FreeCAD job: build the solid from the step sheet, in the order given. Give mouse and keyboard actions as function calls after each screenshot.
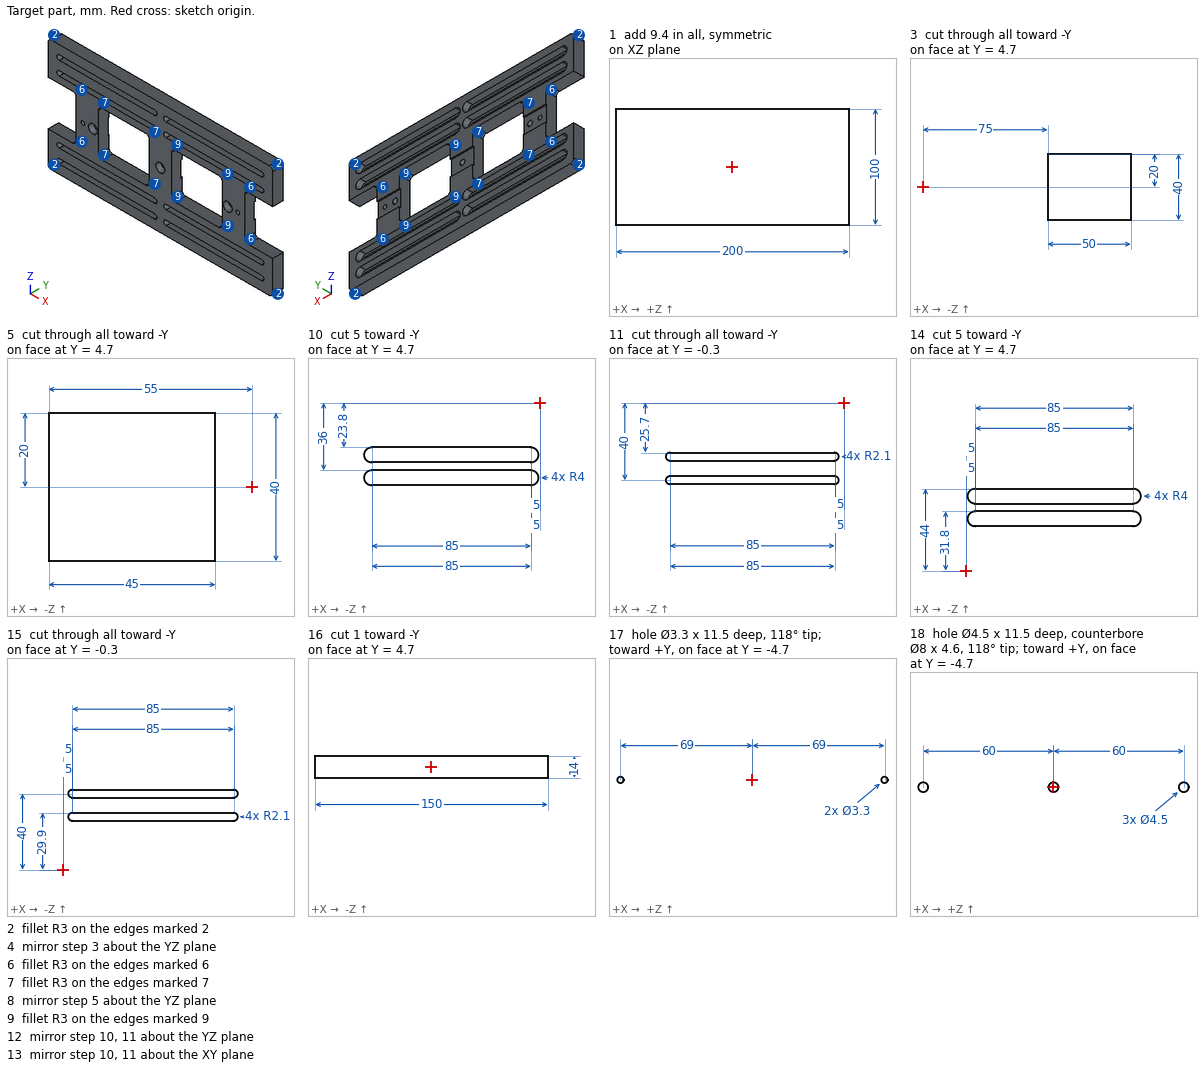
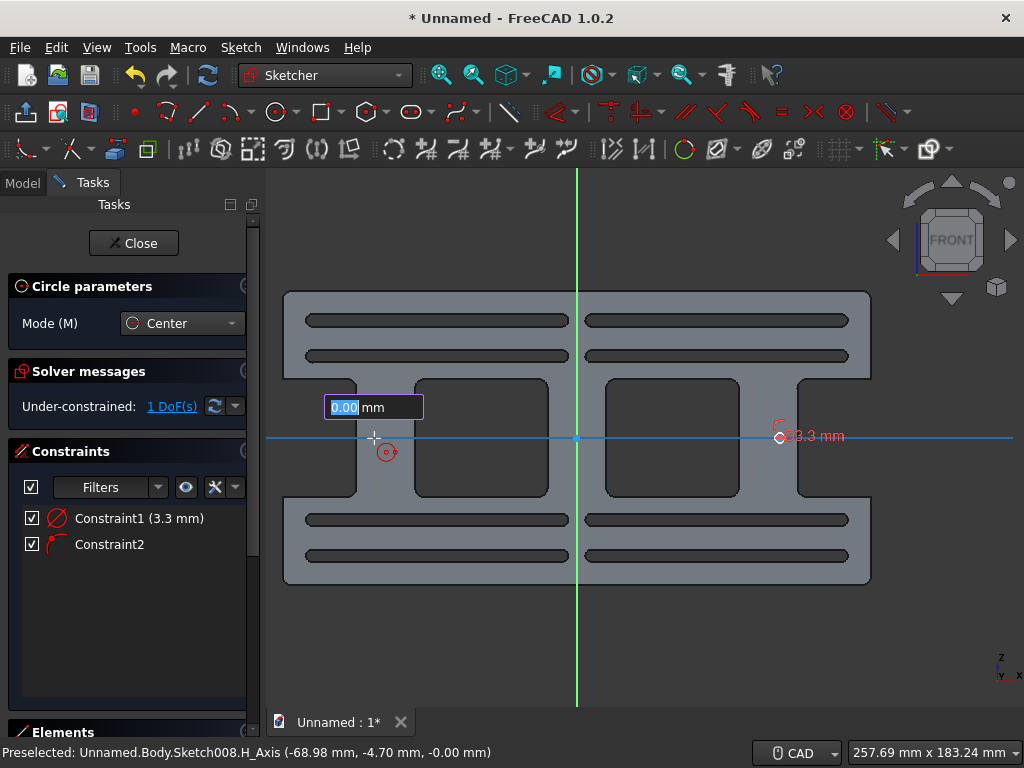
scroll(372, 443, up, 7)
move(373, 440)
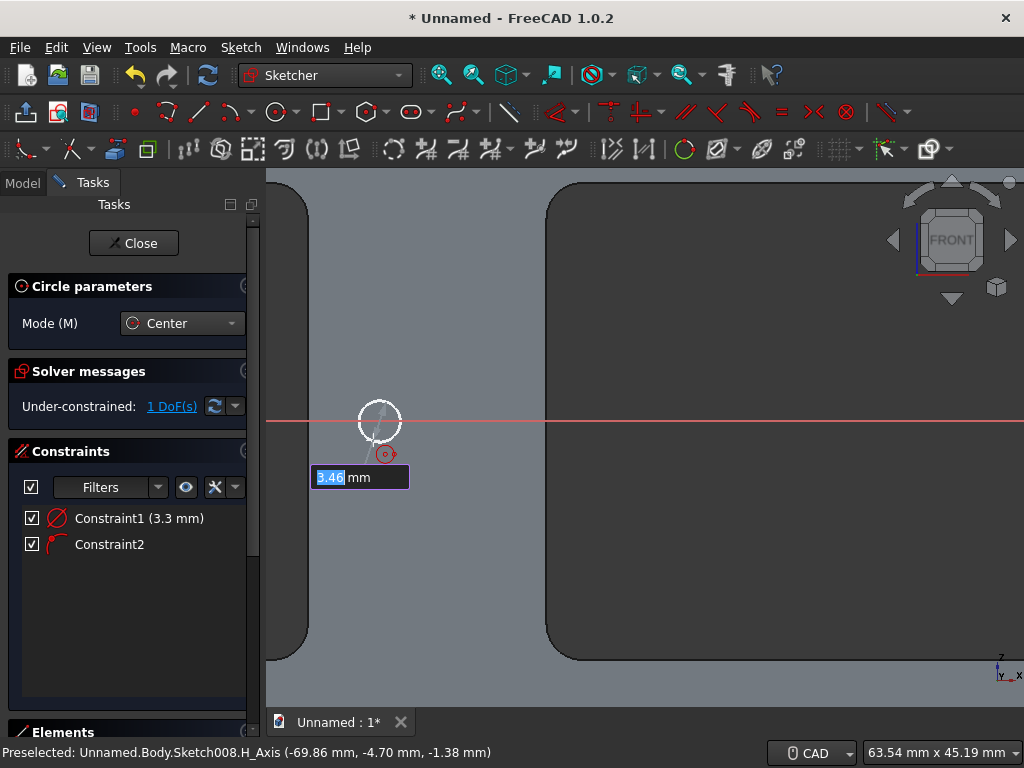
text(3.3)
key(Return)
key(Escape)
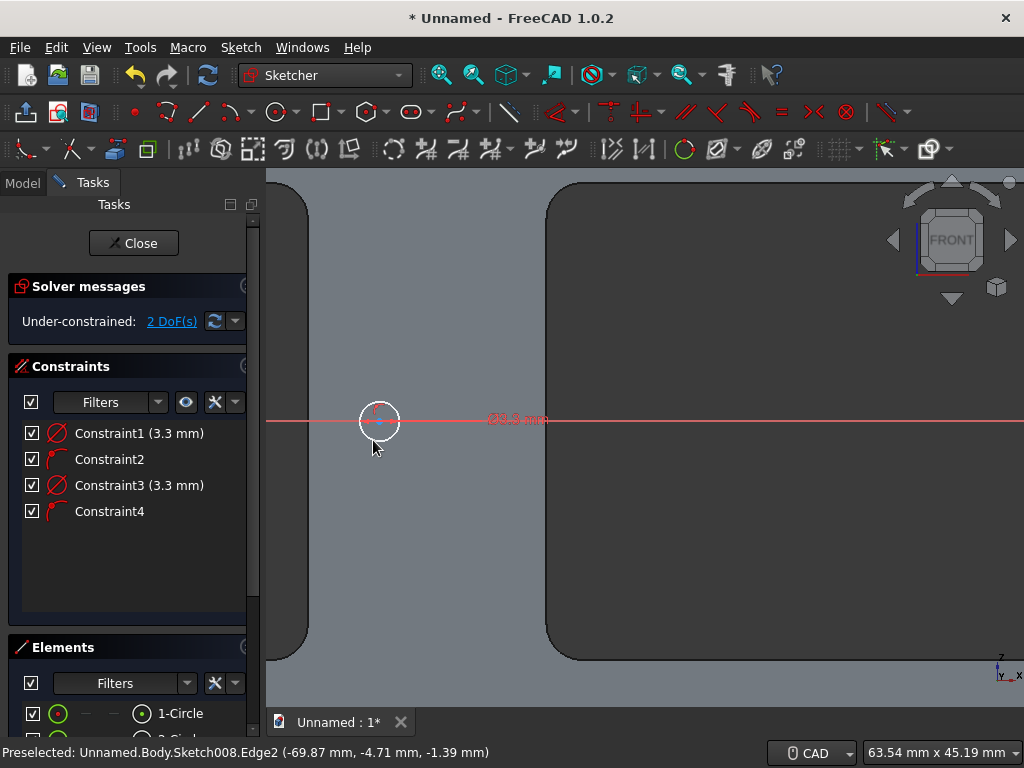
key(d)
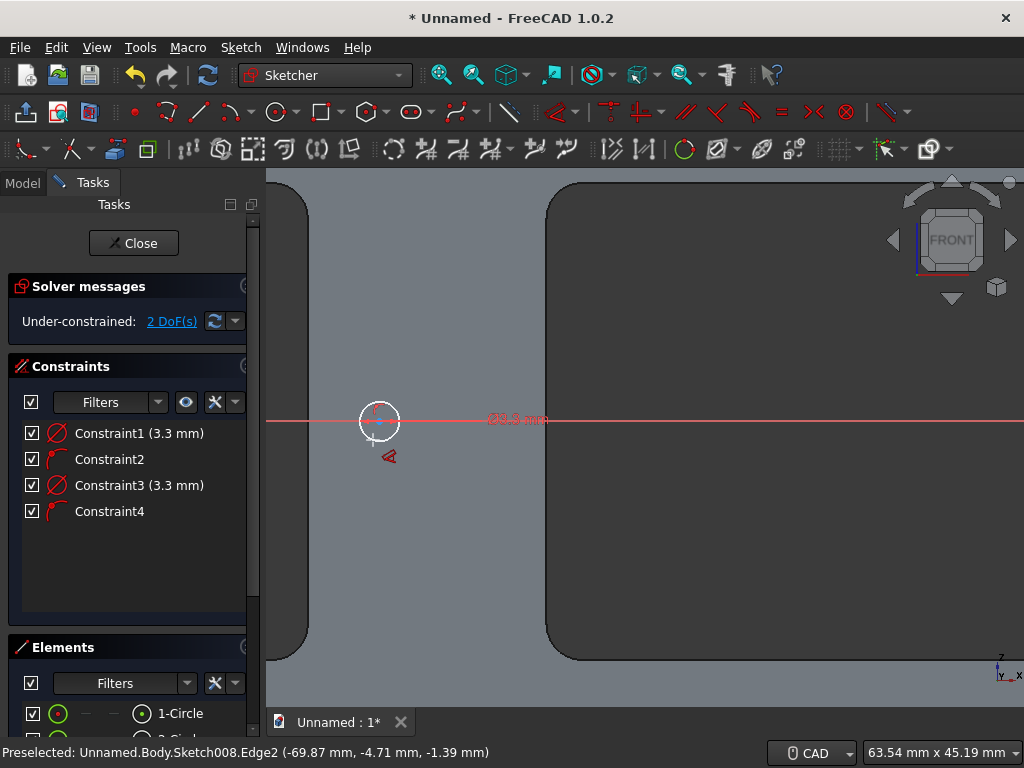
scroll(372, 443, down, 7)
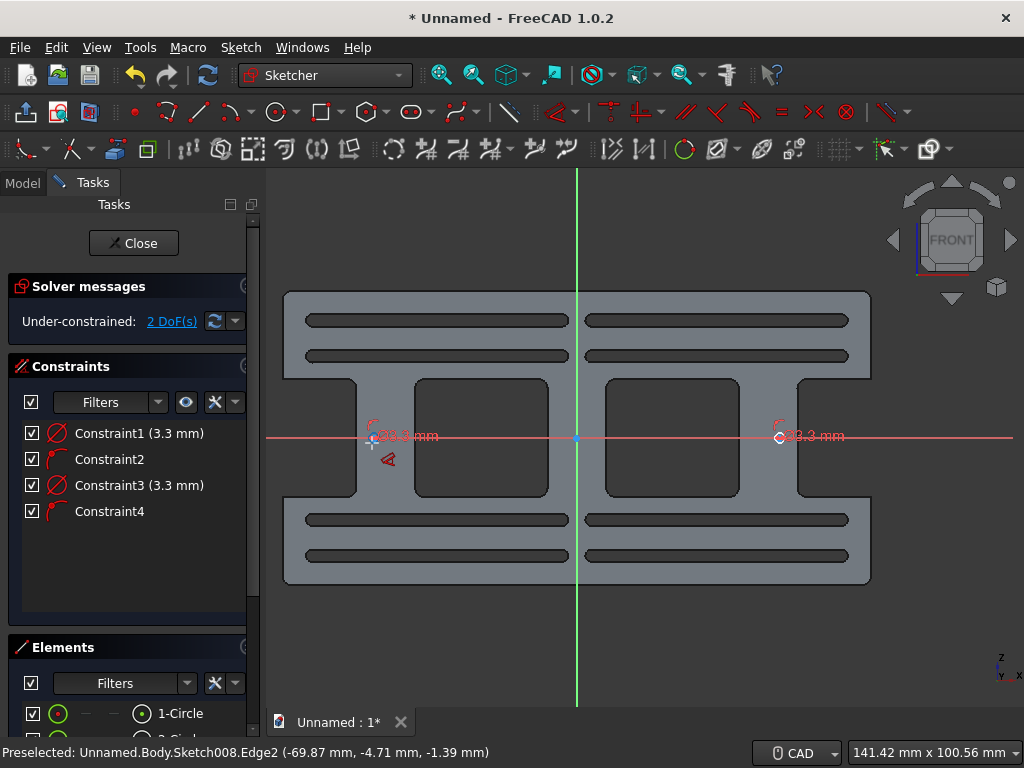
click(780, 438)
click(678, 472)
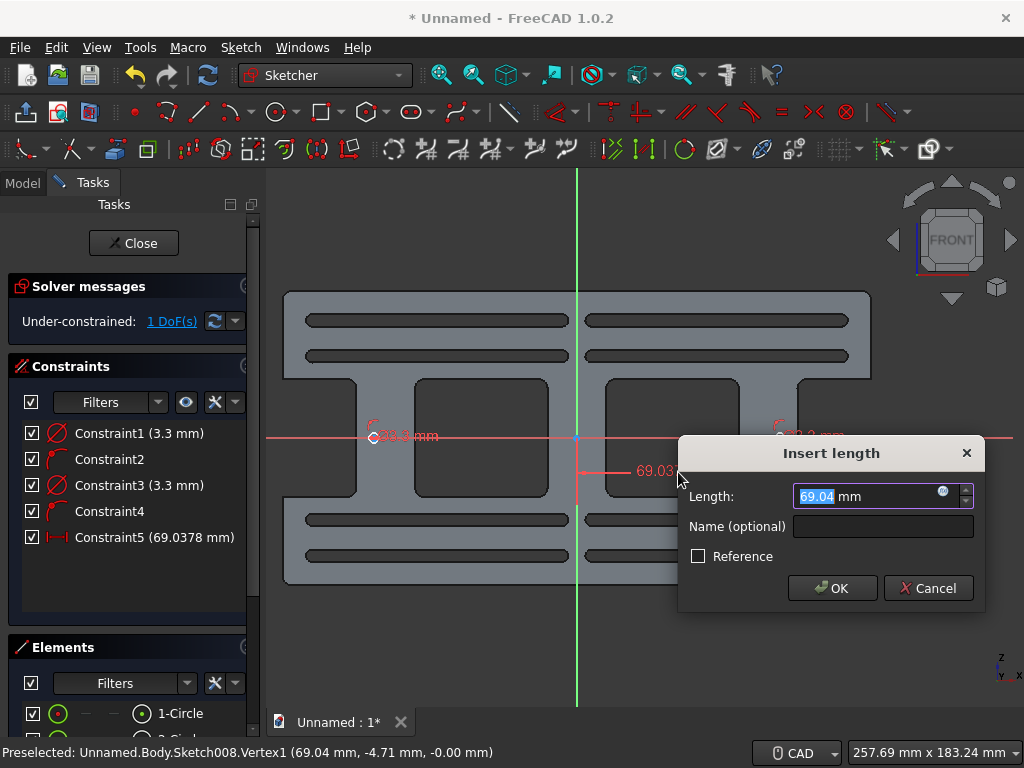
text(69)
key(Return)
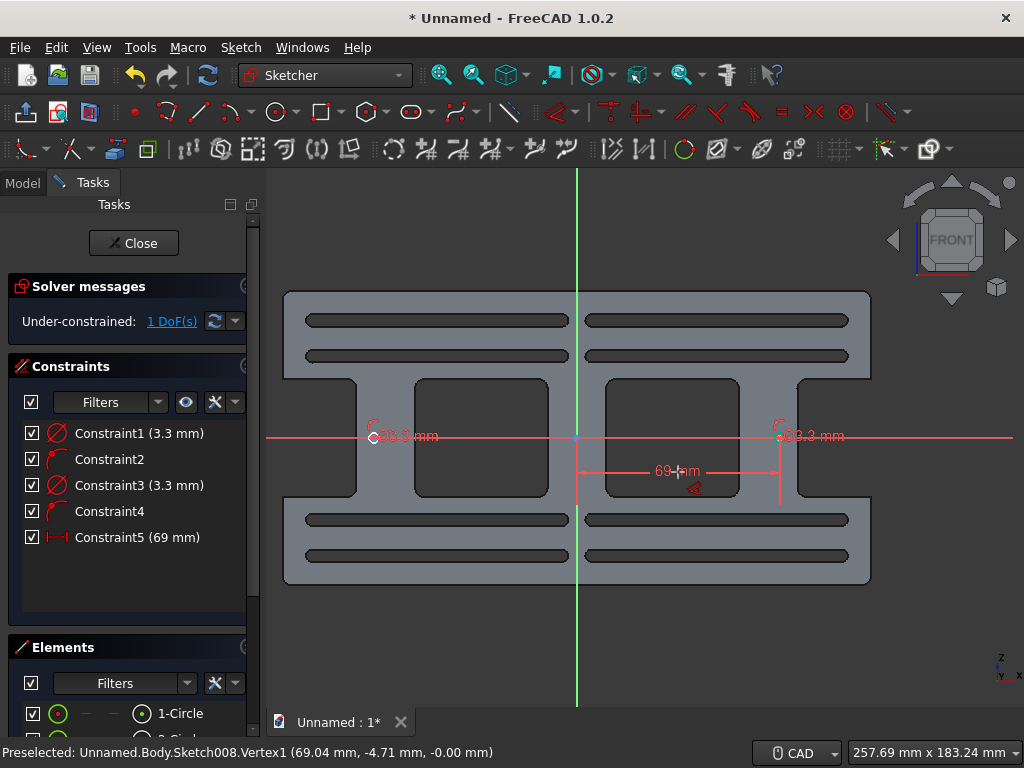
click(374, 438)
click(475, 472)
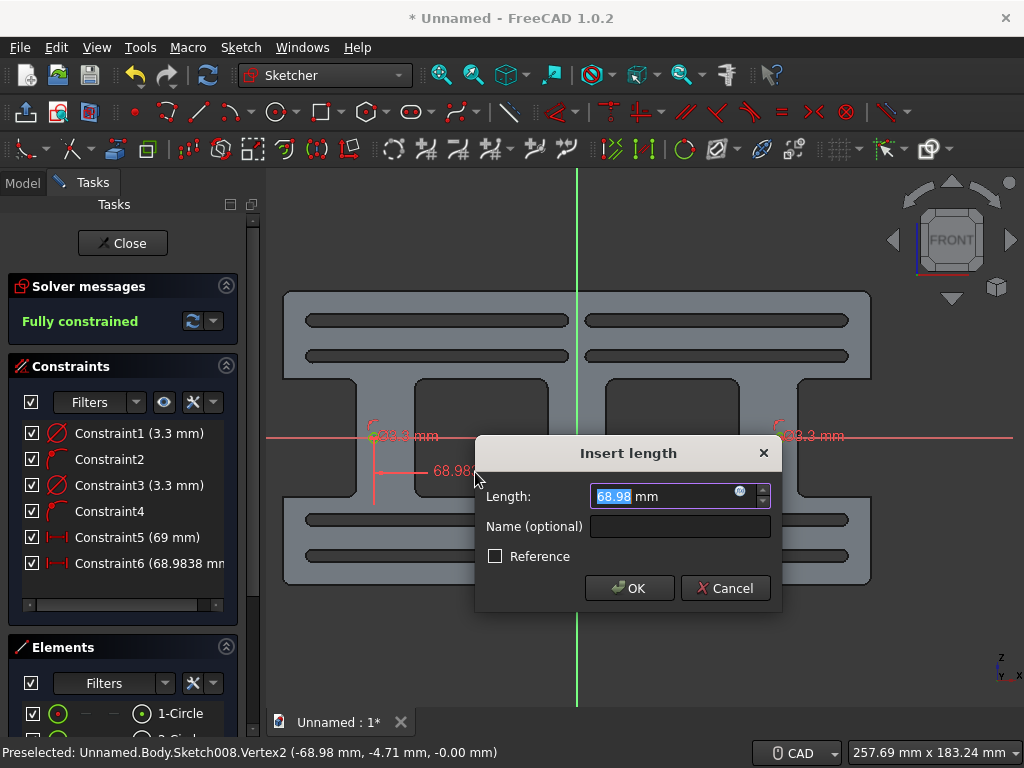
text(69)
key(Return)
key(Escape)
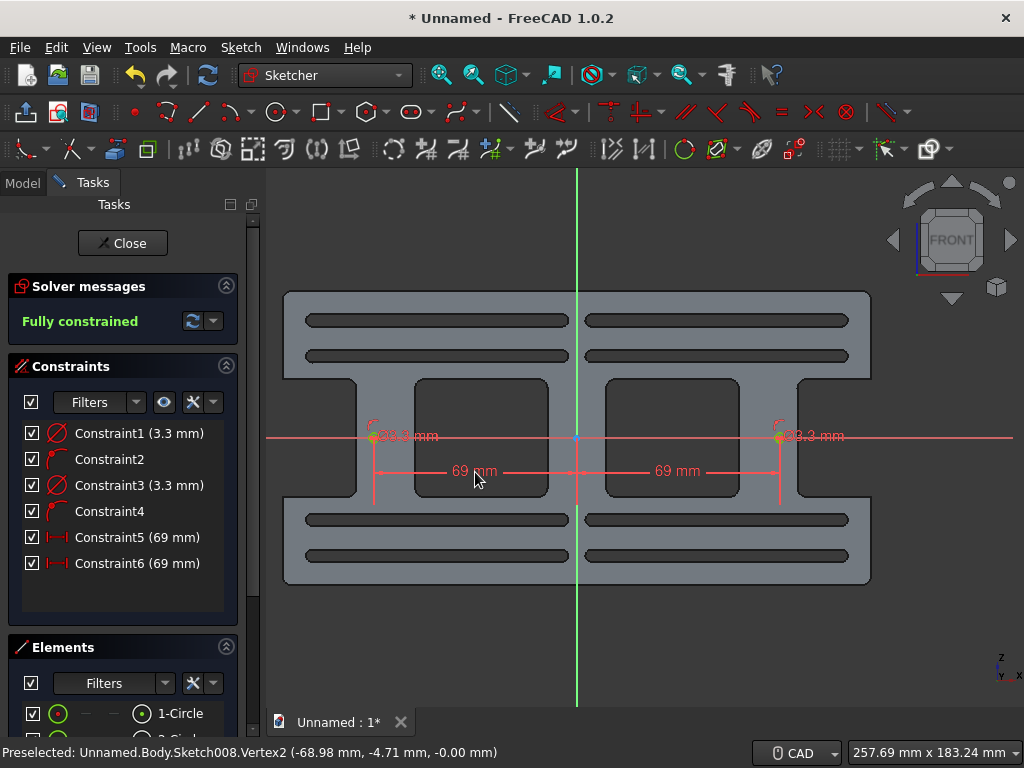
click(123, 243)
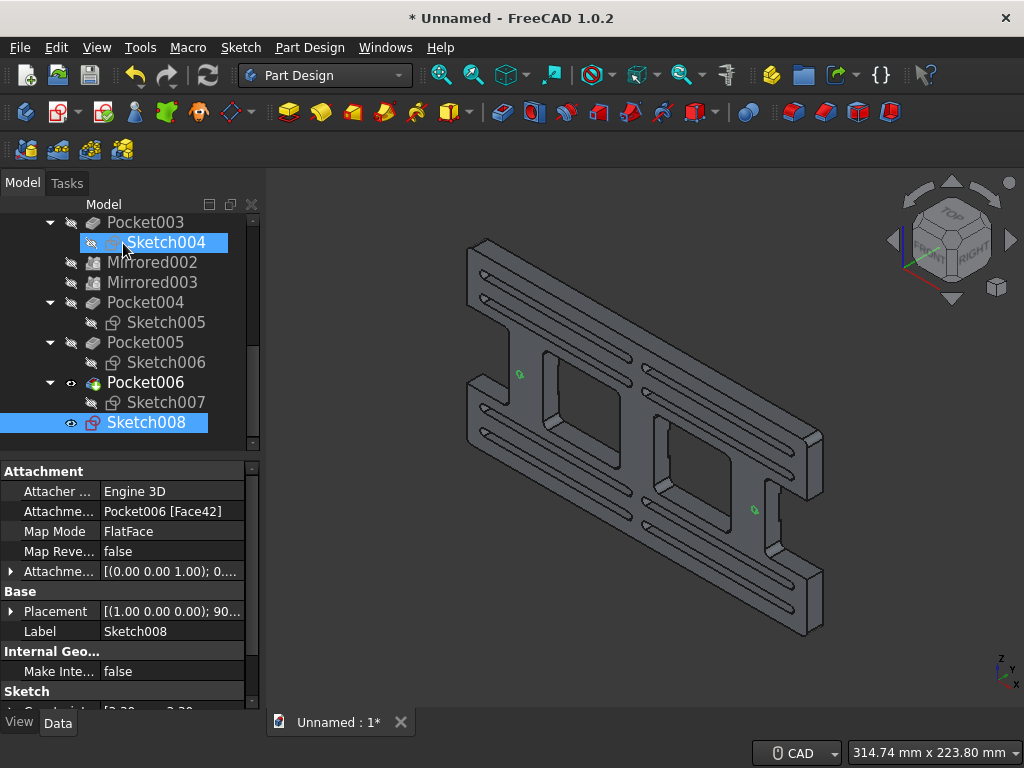
click(536, 112)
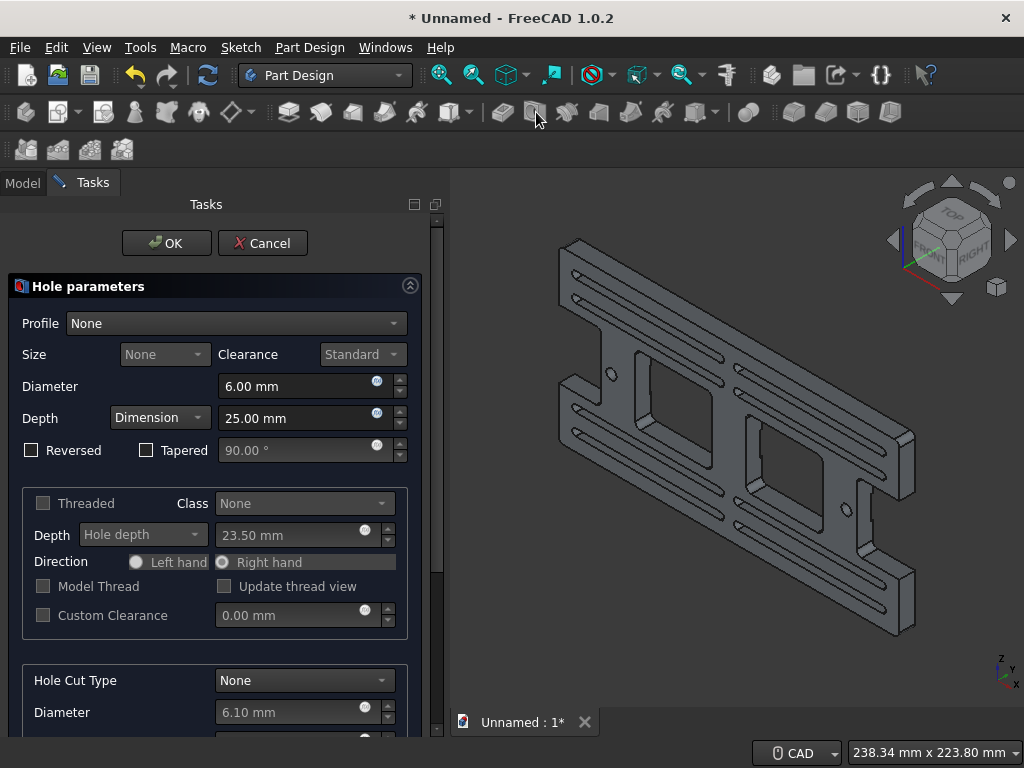
triple_click(305, 386)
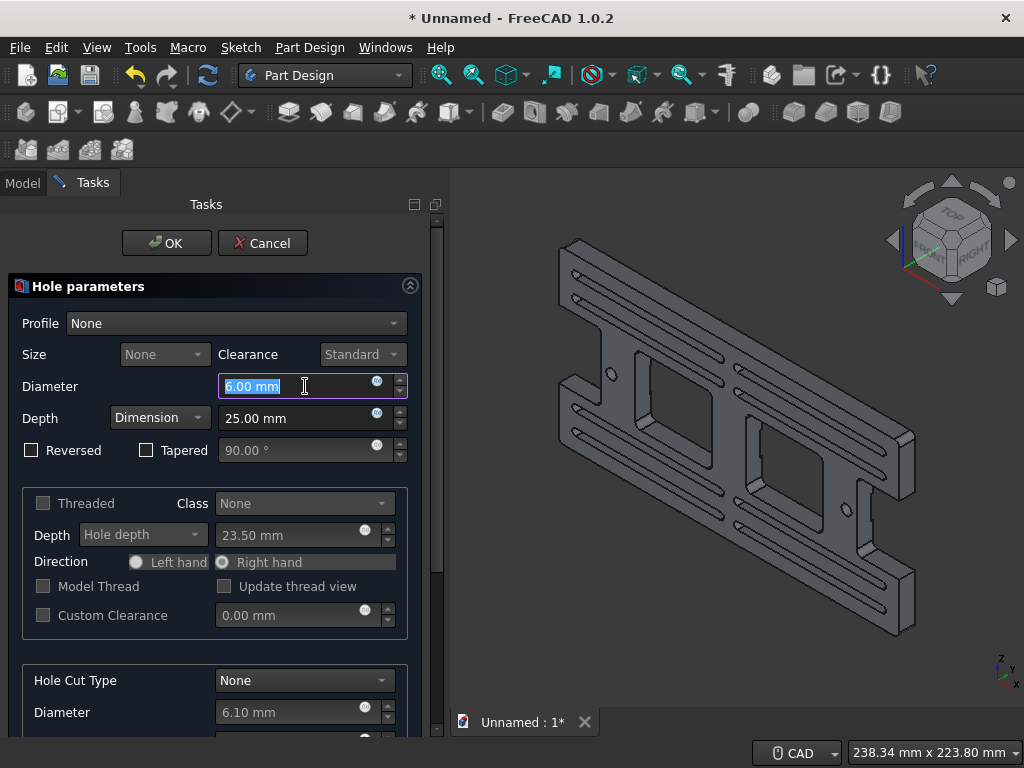
text(3.3)
key(Tab)